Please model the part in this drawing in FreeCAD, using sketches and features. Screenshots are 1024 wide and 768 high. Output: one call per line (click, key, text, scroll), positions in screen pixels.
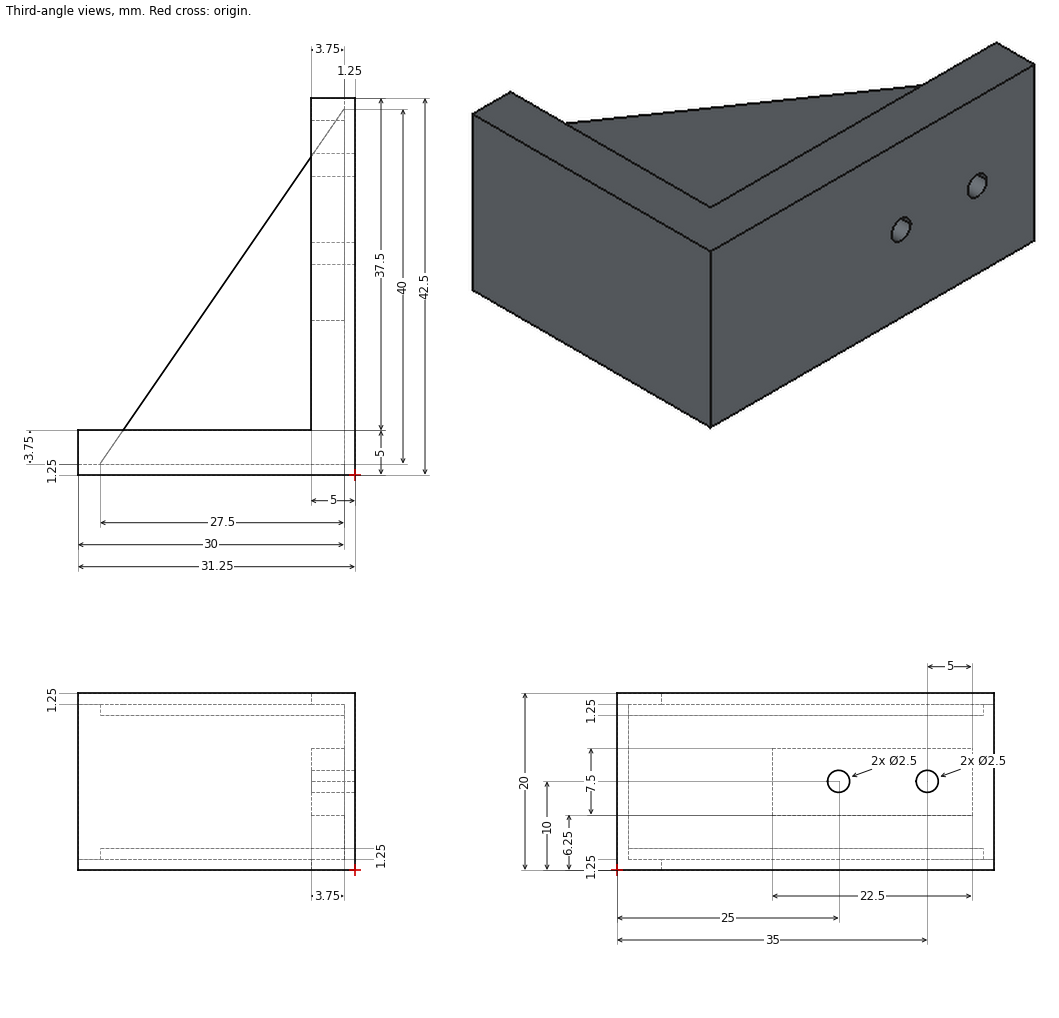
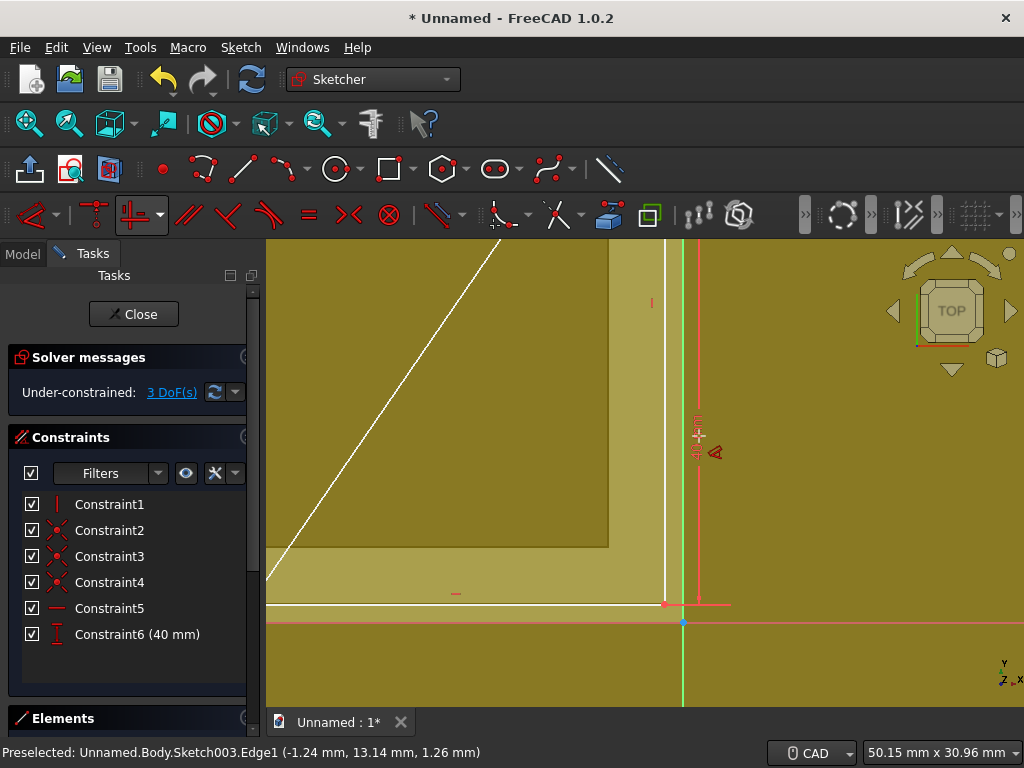
click(374, 605)
click(479, 639)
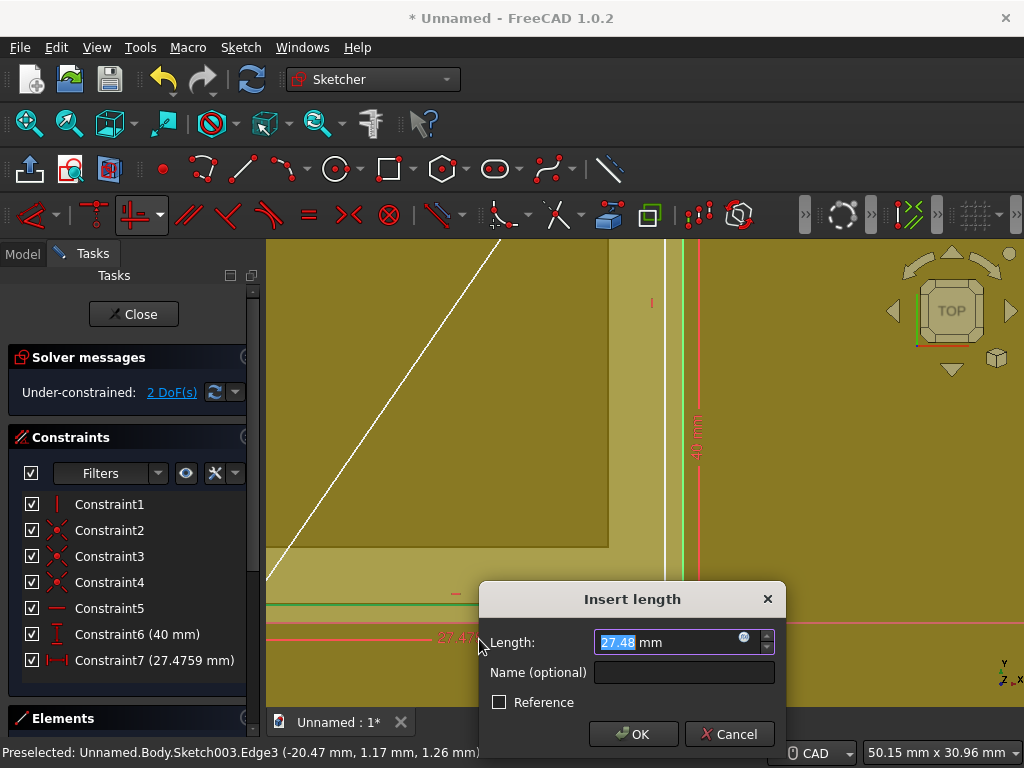
text(27.5)
key(Return)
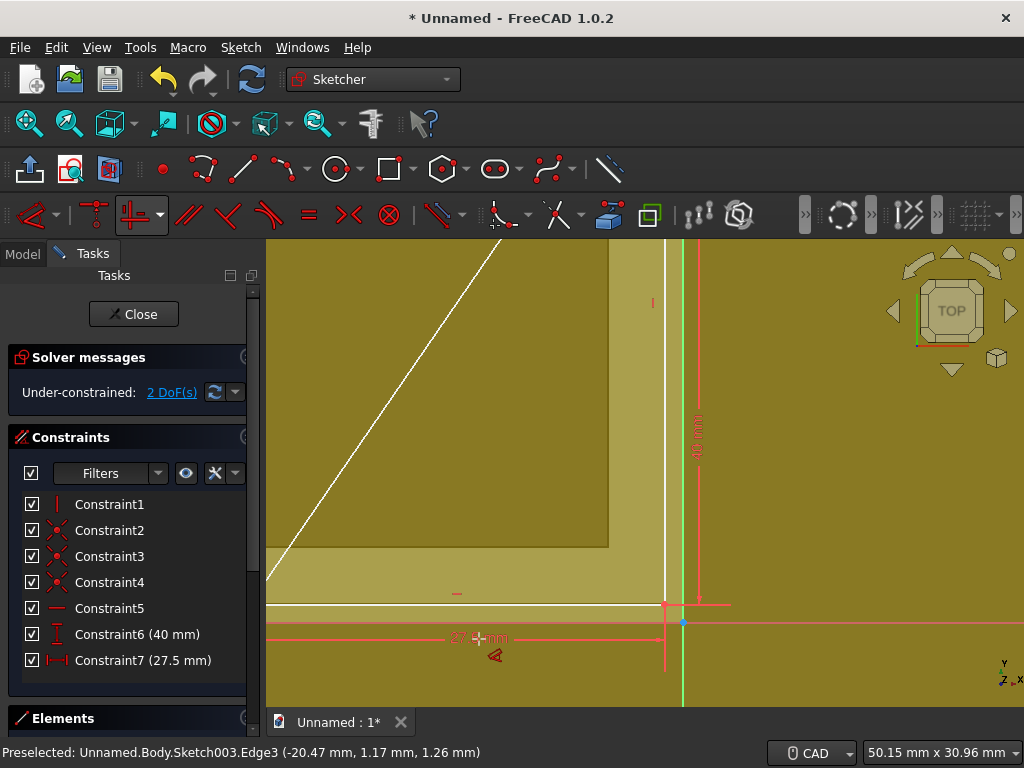
scroll(665, 605, up, 4)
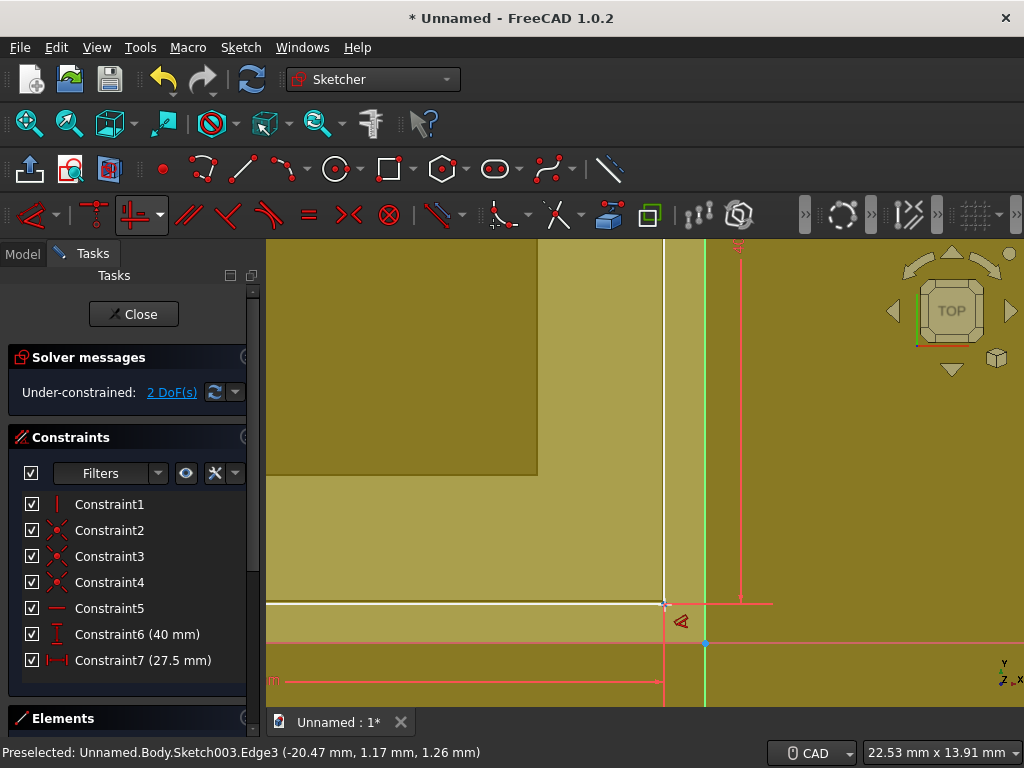
click(664, 604)
click(685, 677)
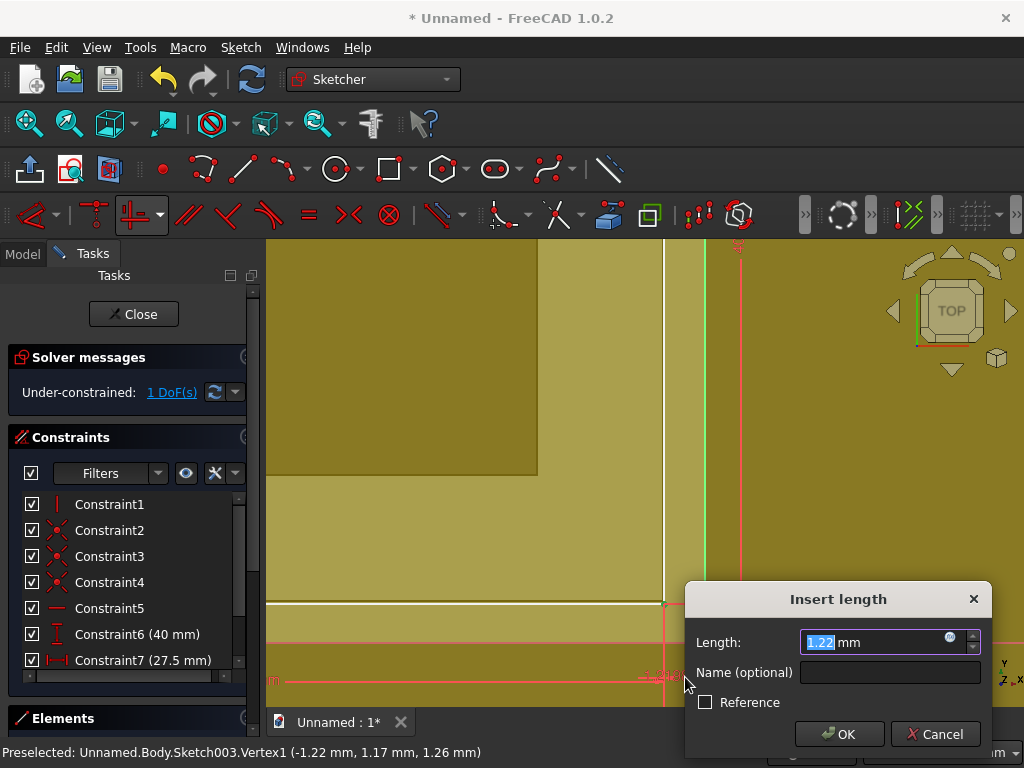
text(1.25)
key(Return)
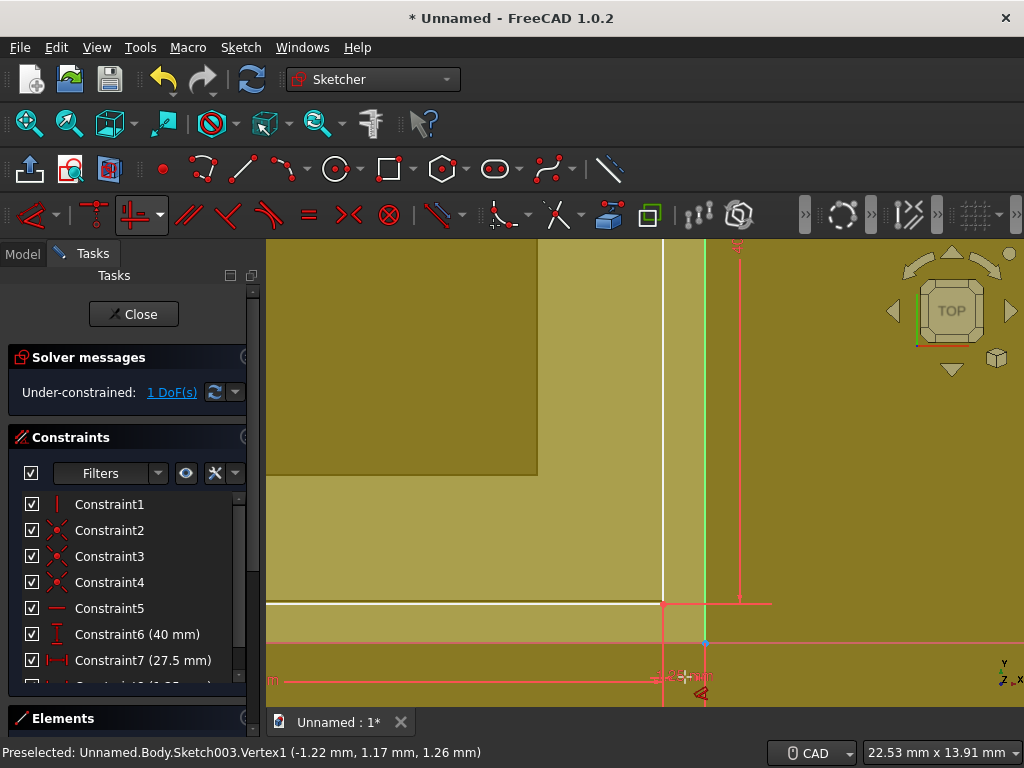
click(663, 604)
click(739, 624)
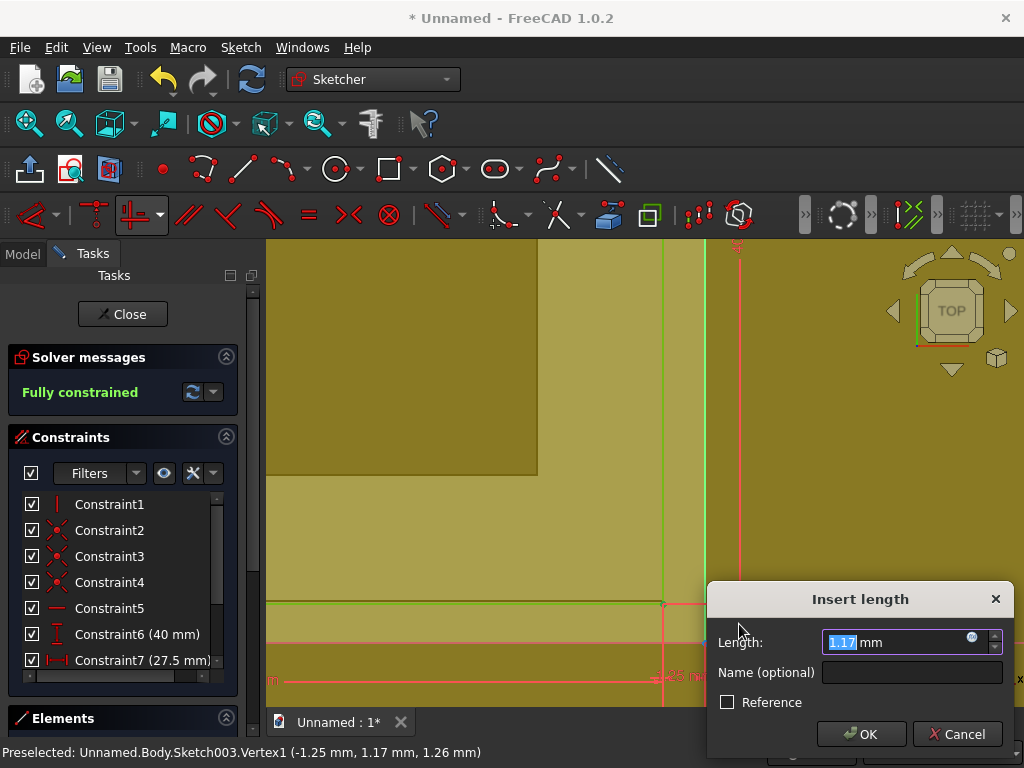
text(1.25)
key(Return)
key(Escape)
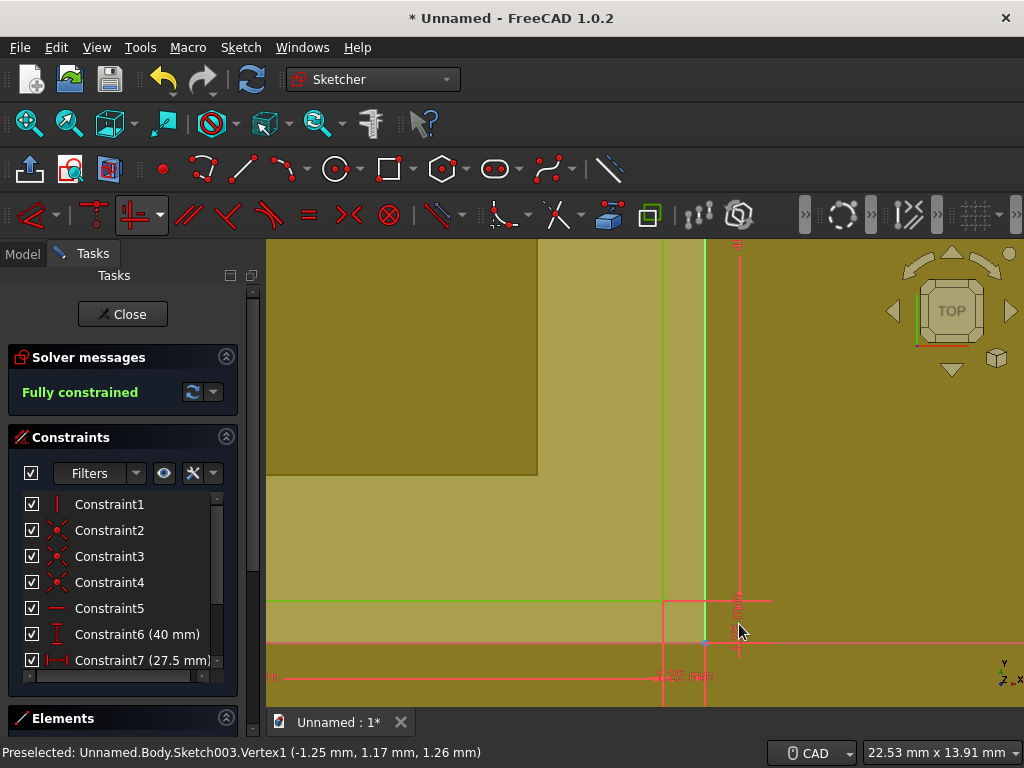
click(123, 314)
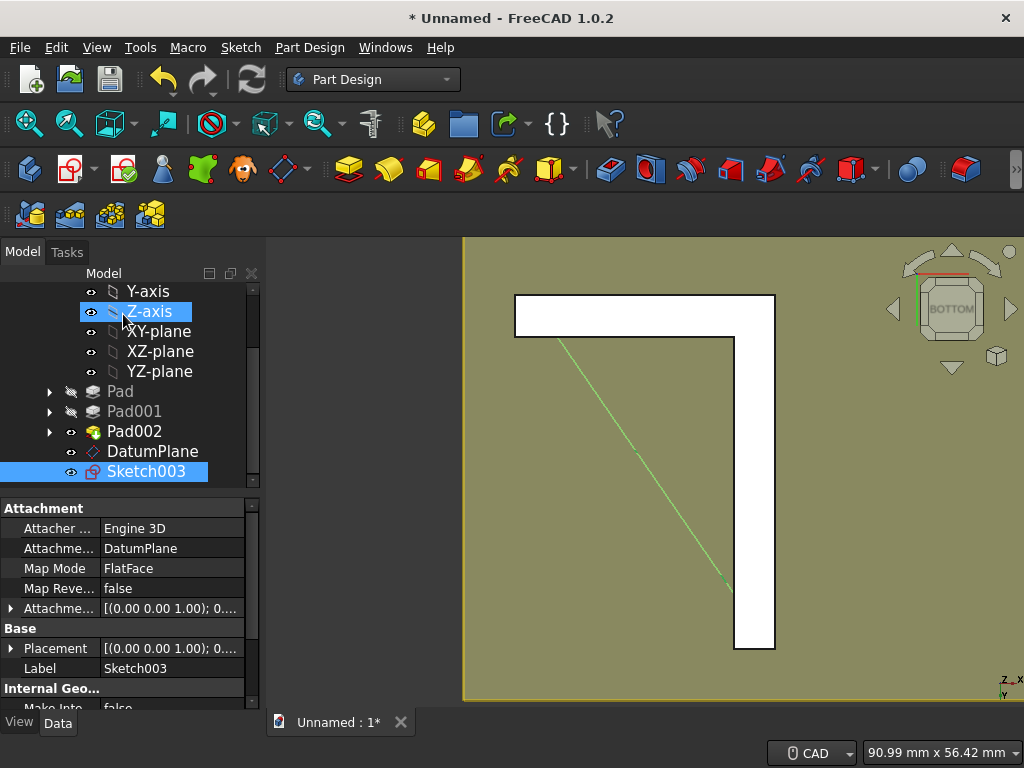
click(350, 170)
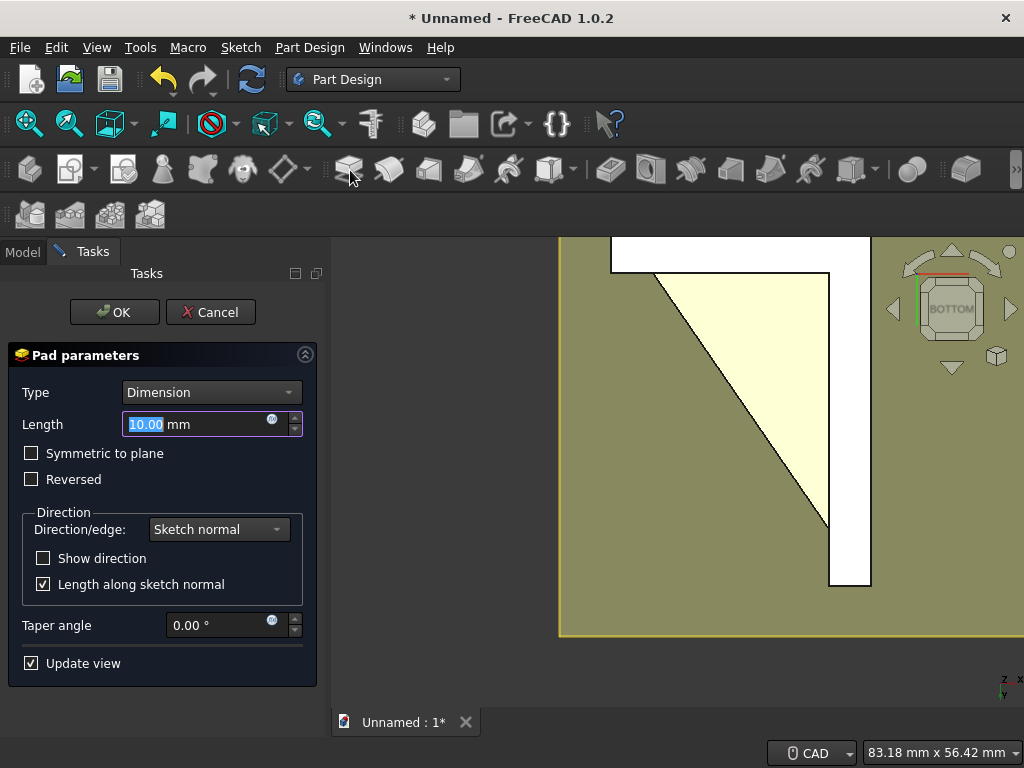
text(1.25)
key(Tab)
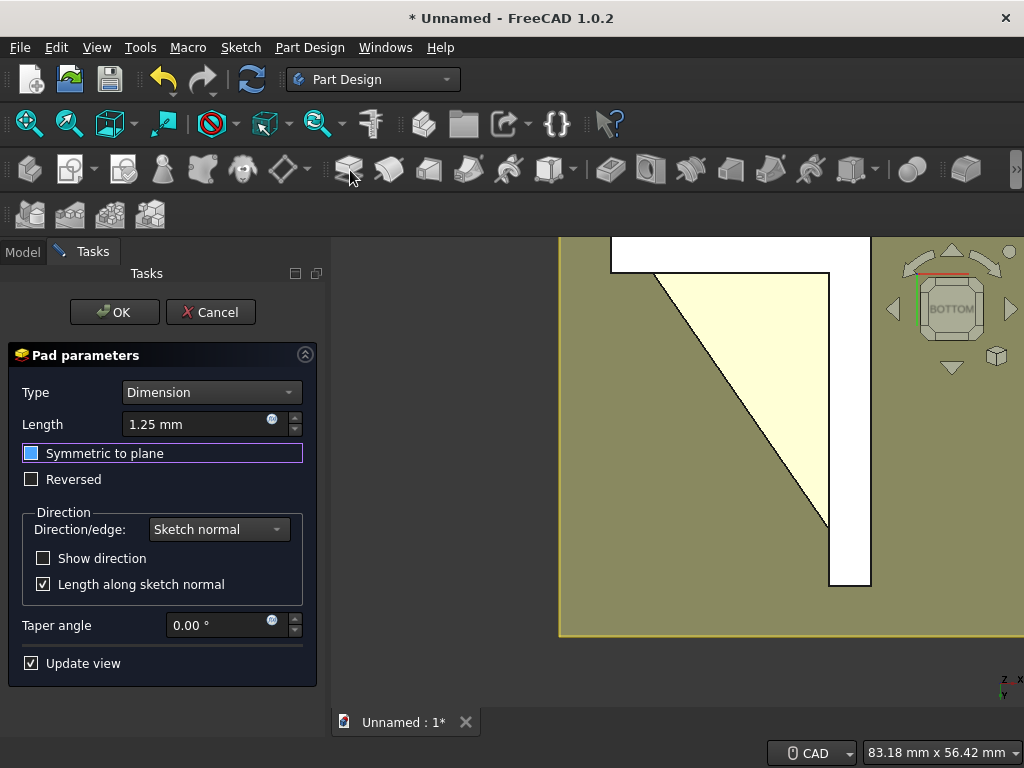
click(115, 312)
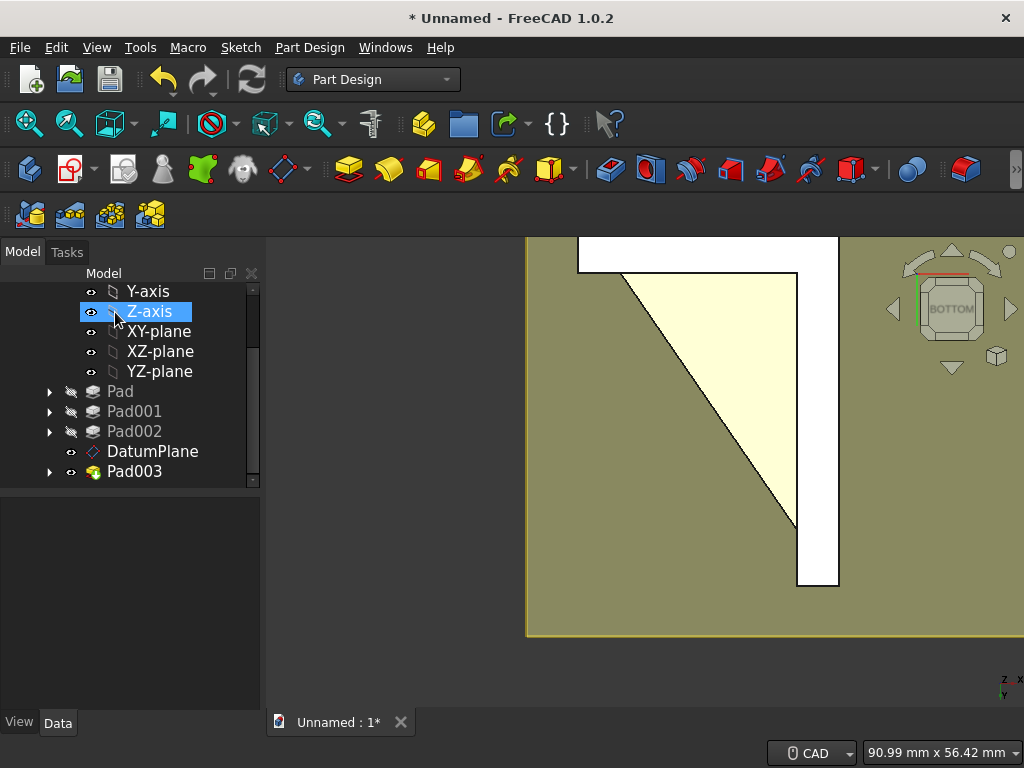
click(116, 452)
key(space)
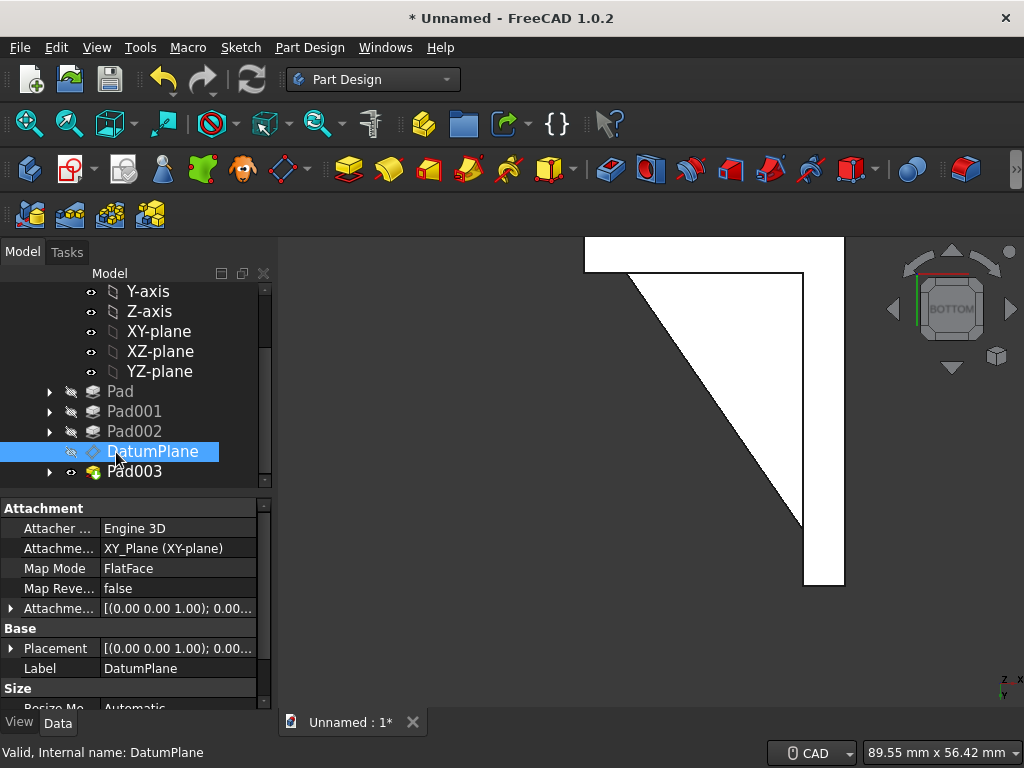
key(v)
key(f)